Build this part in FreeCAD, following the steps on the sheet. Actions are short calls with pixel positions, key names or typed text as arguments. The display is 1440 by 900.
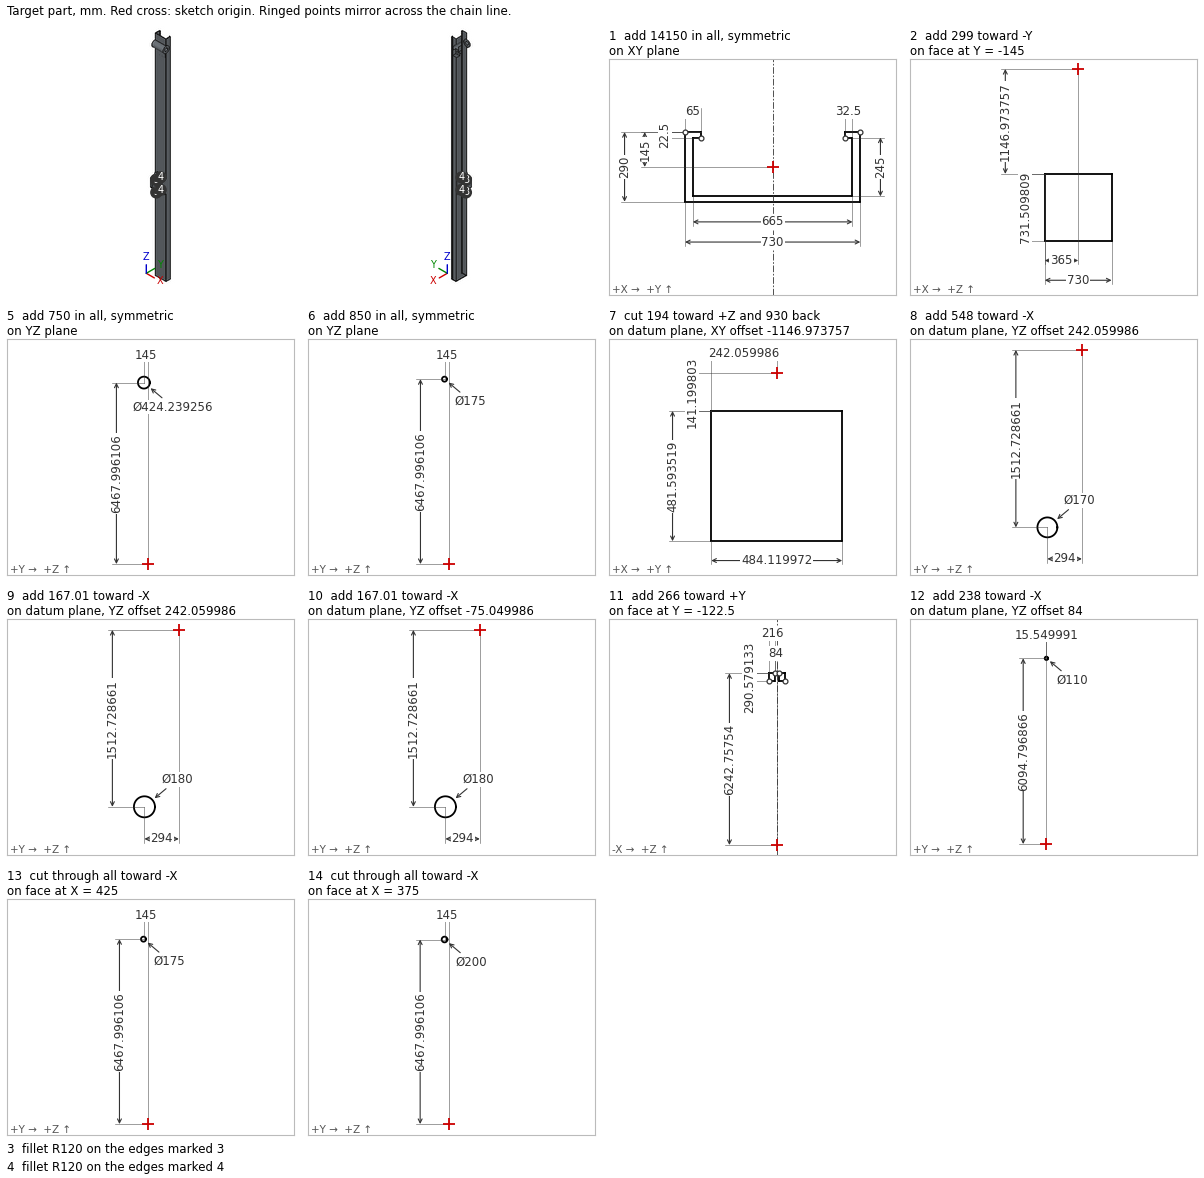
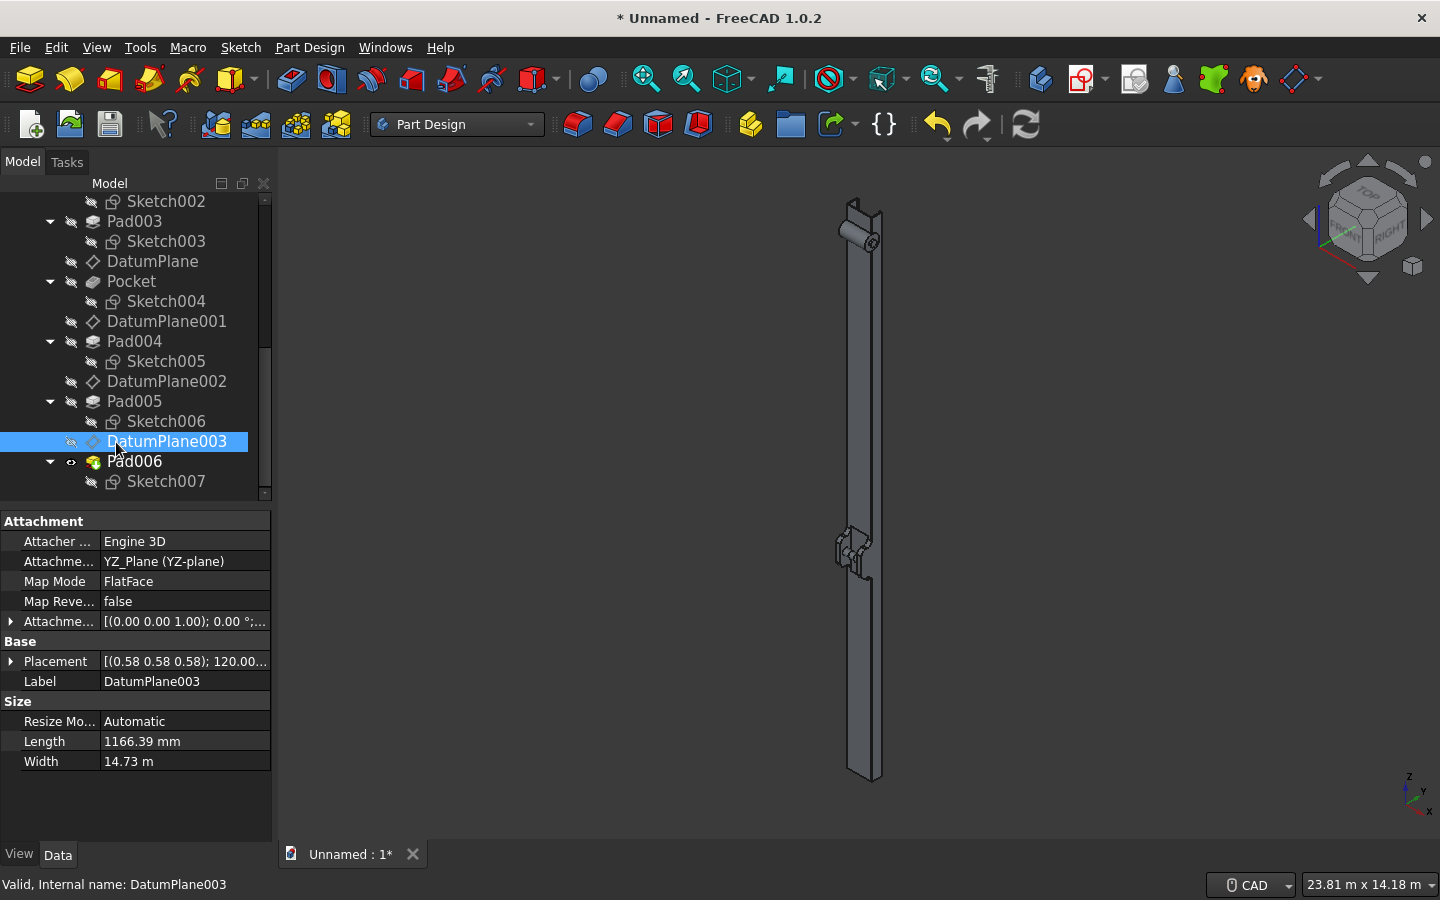
key(4)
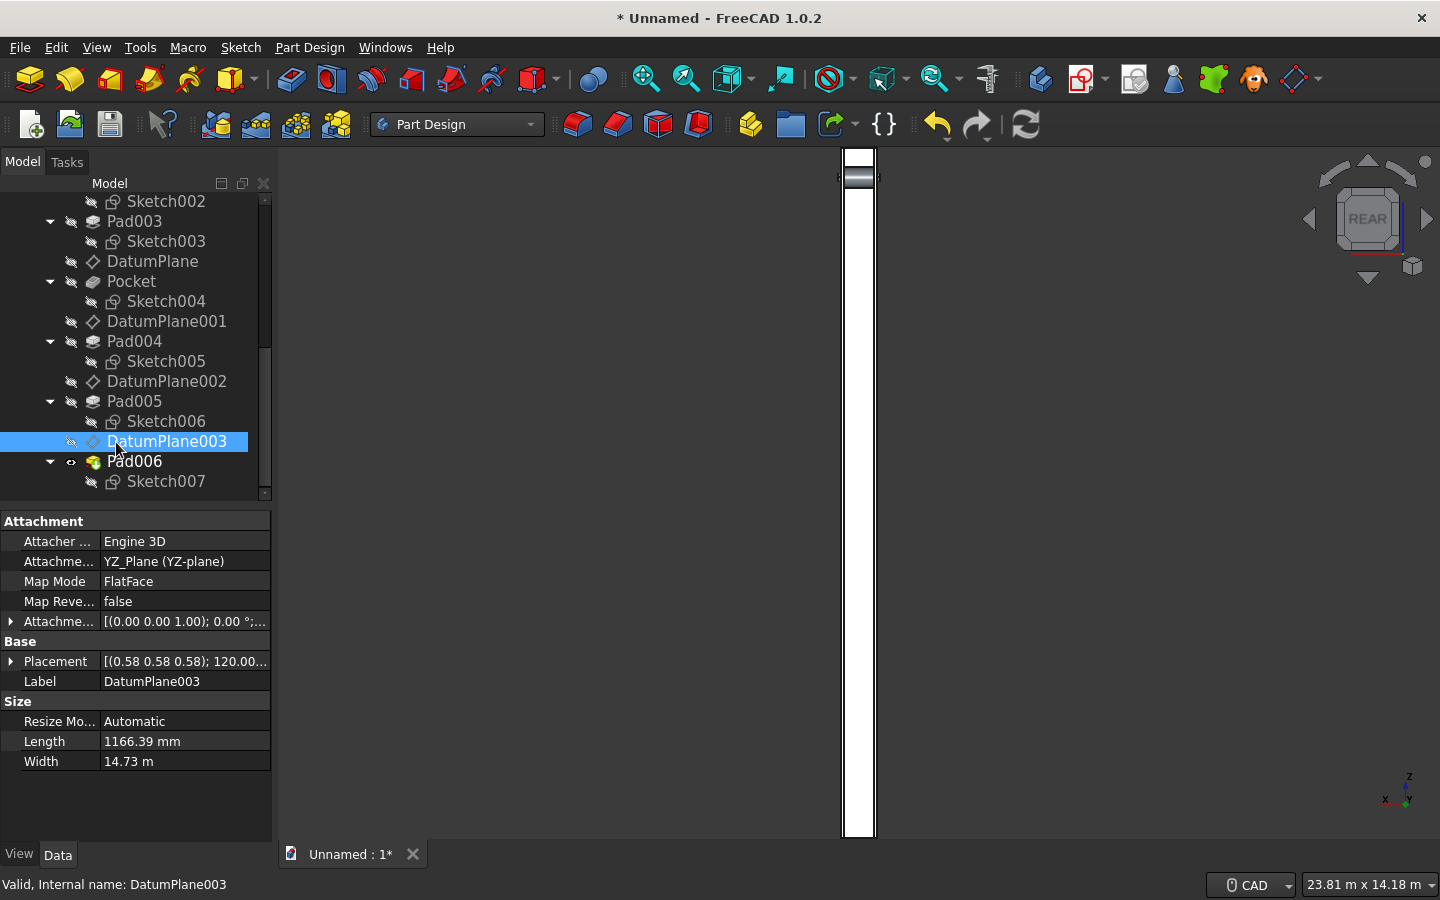
click(859, 233)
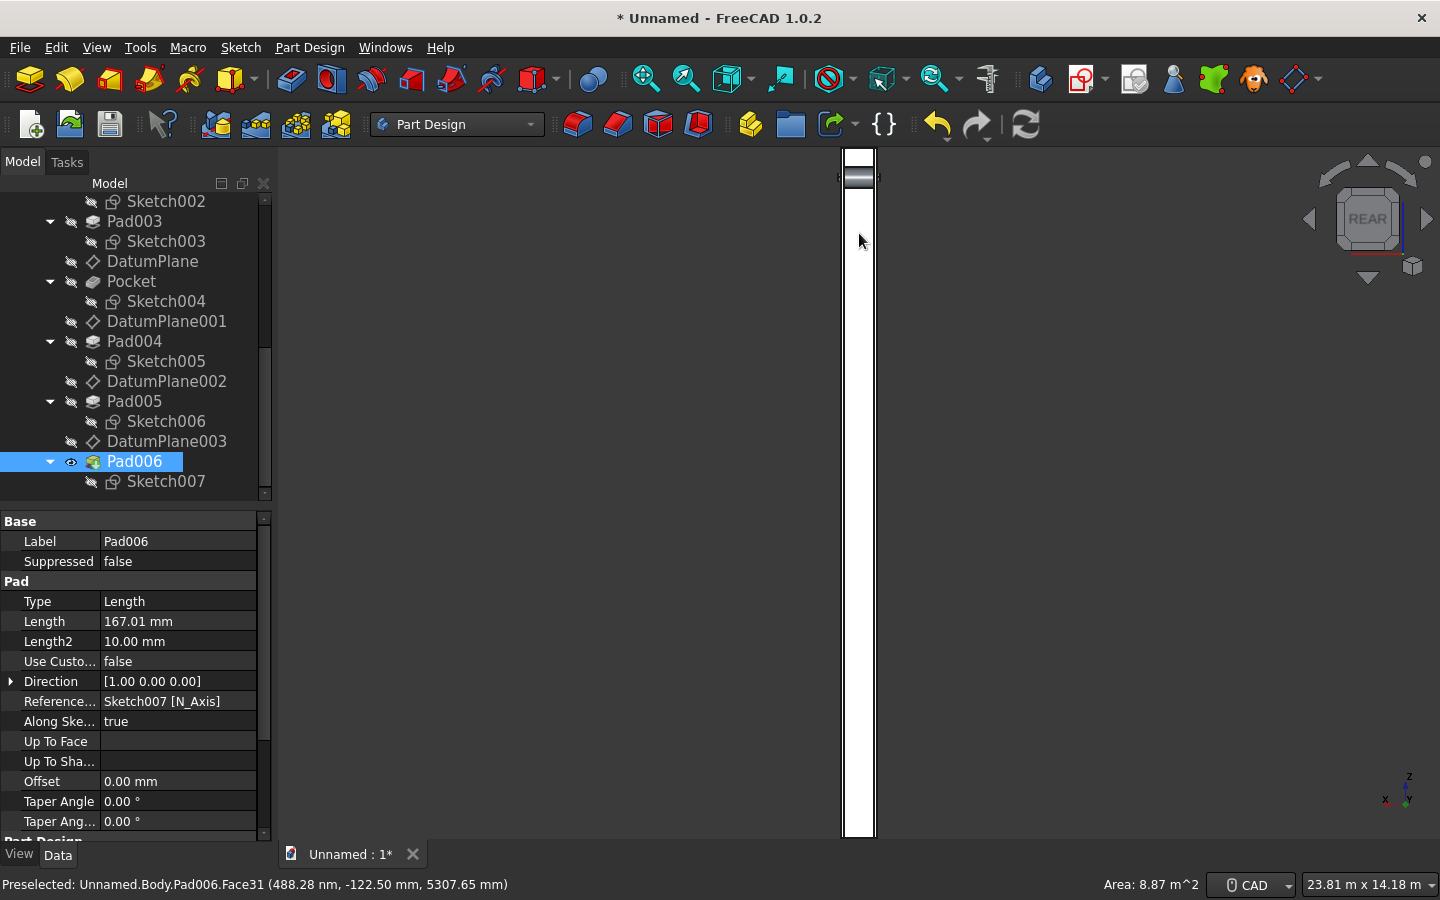
click(1082, 80)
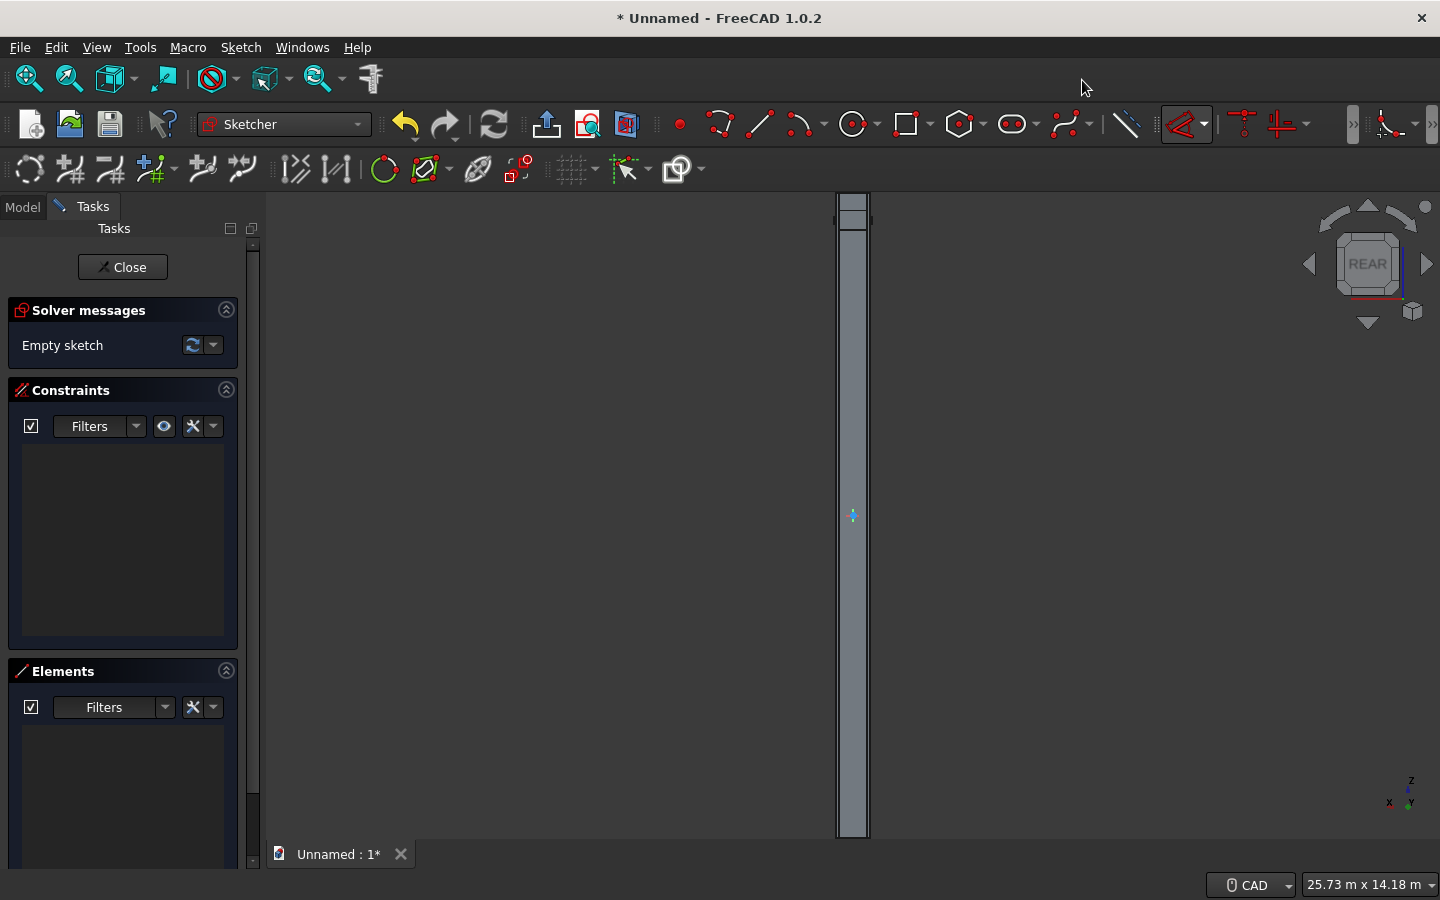
key(q)
key(s)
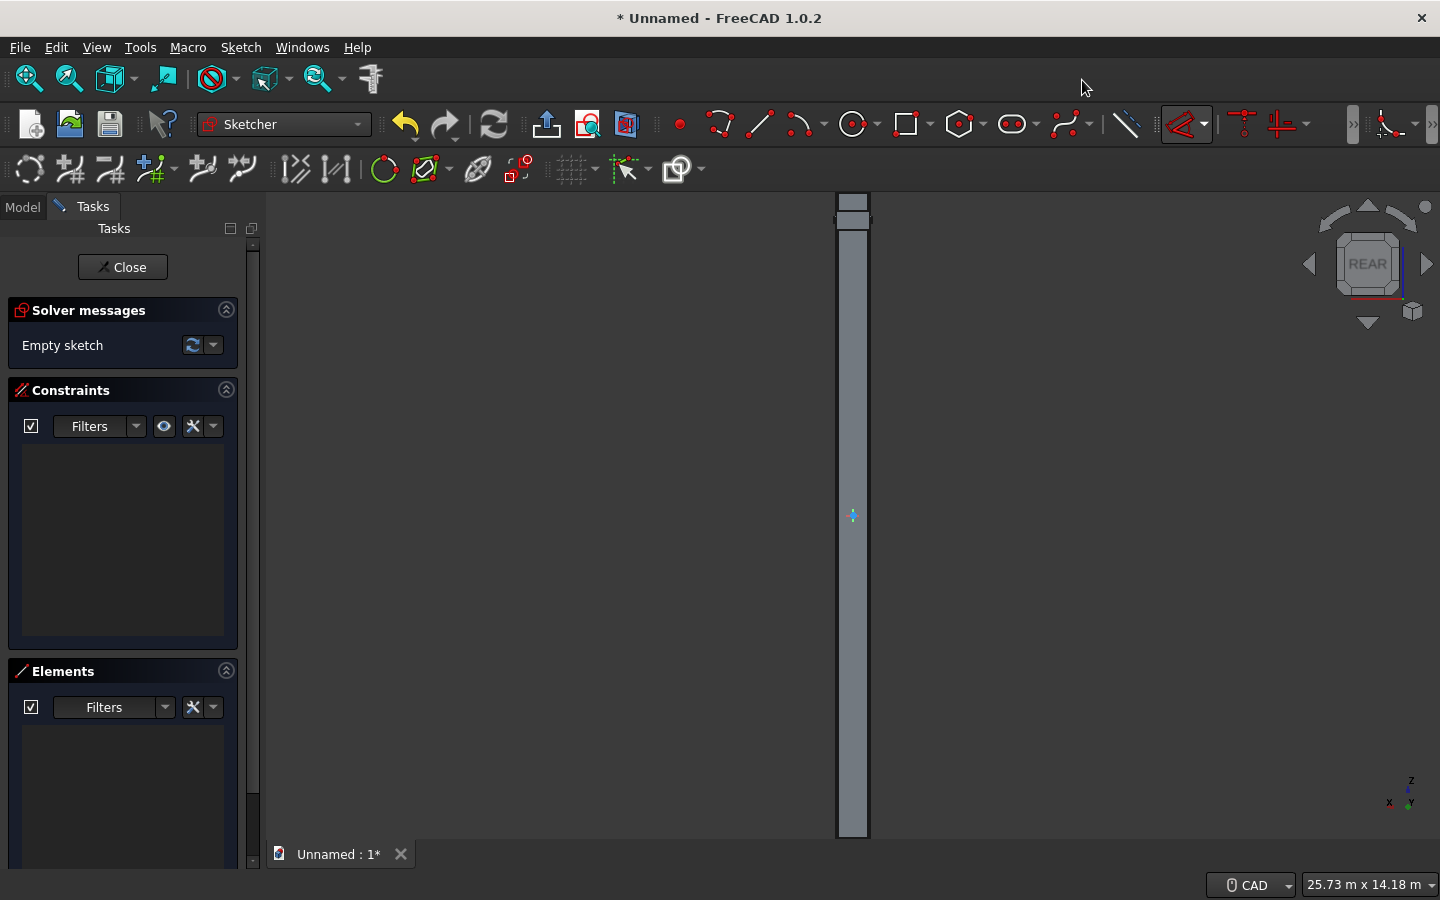
scroll(857, 223, up, 15)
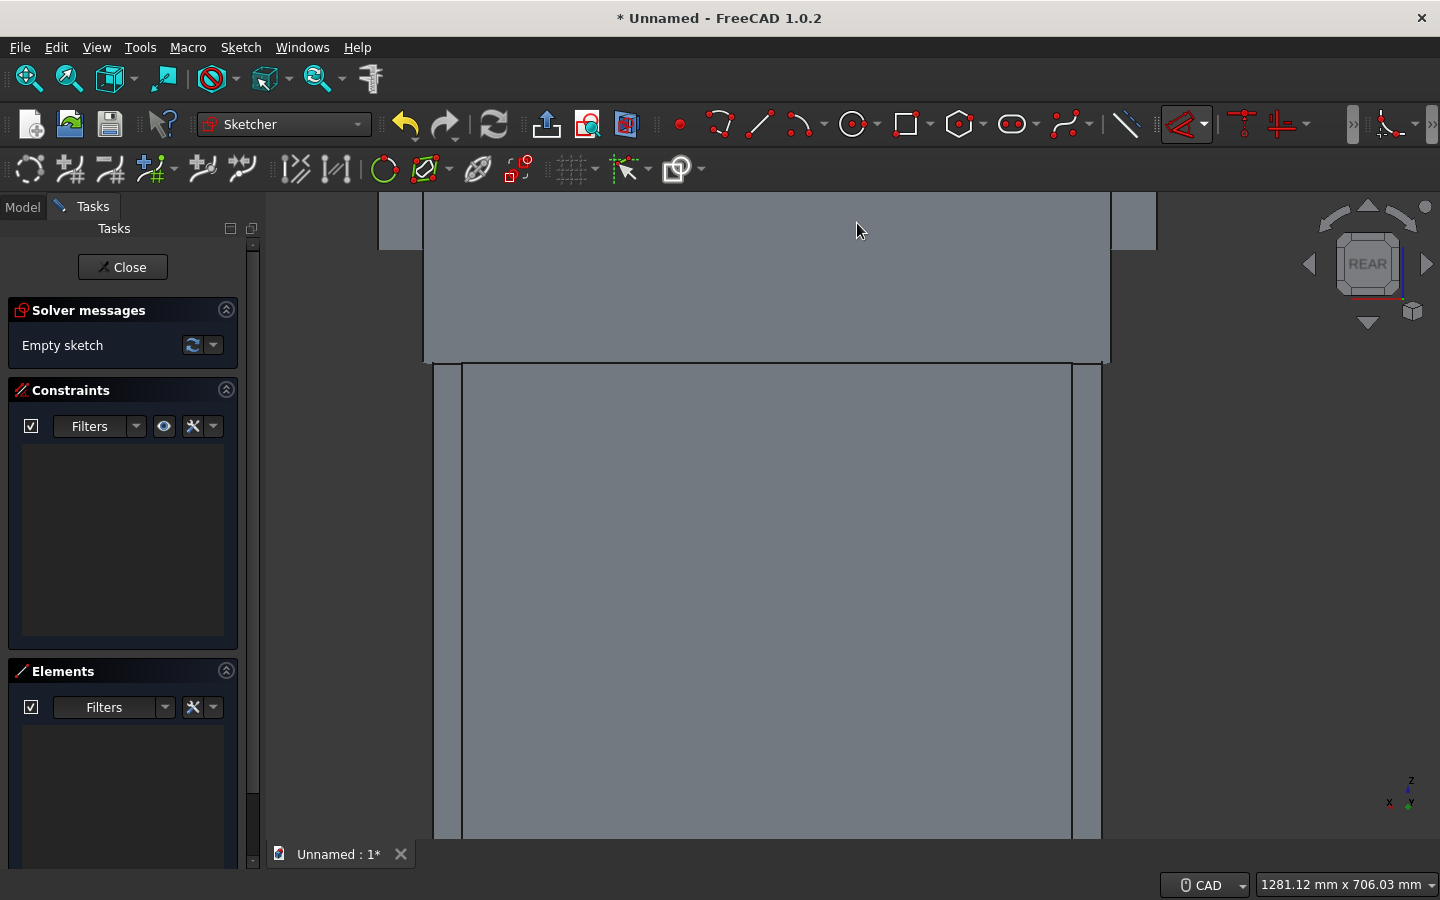
click(906, 124)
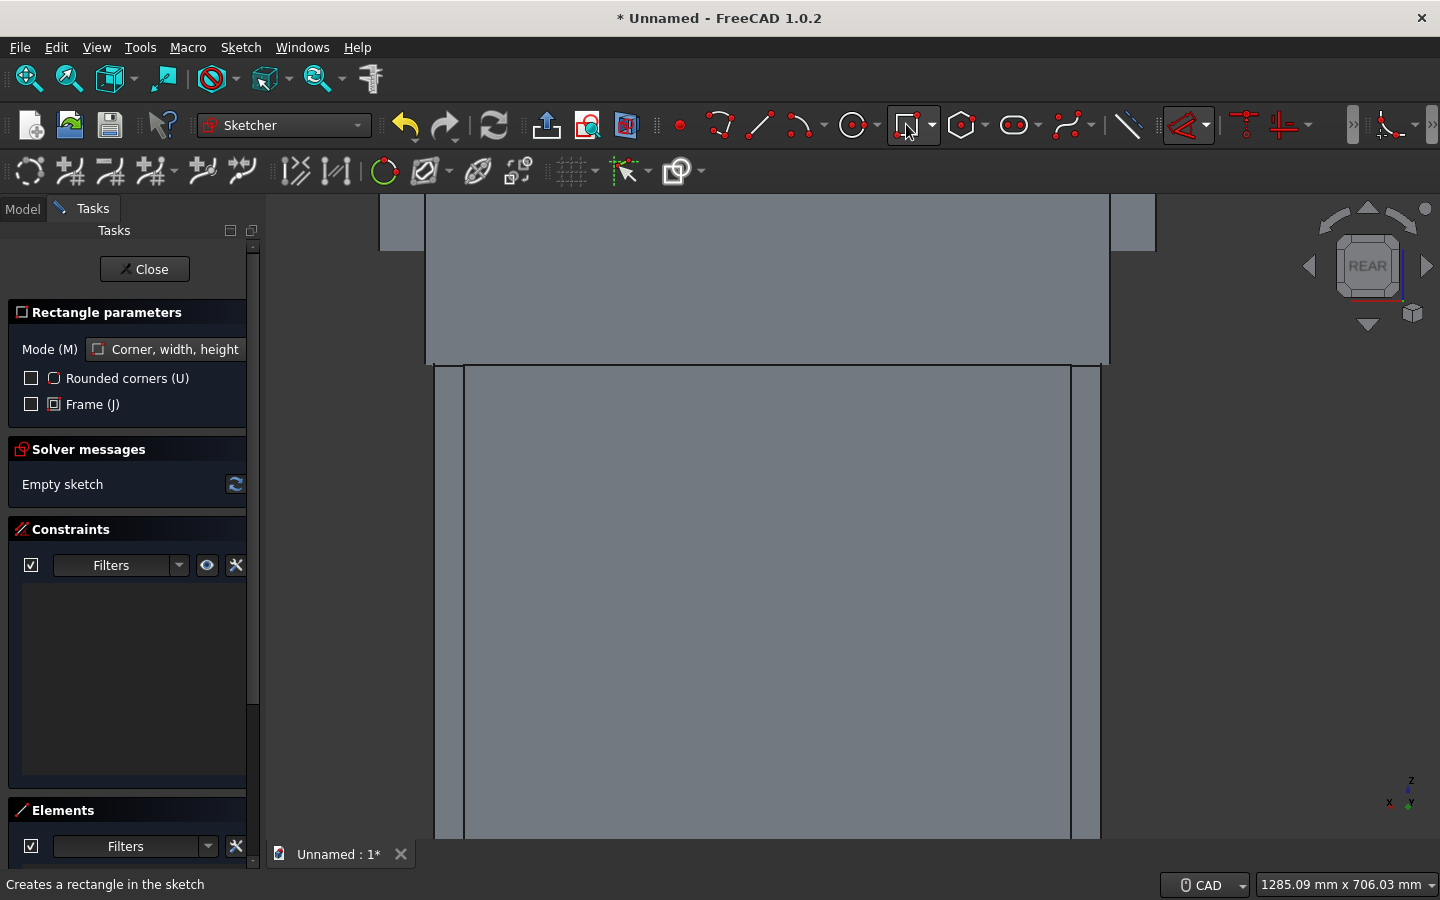
click(493, 378)
click(691, 643)